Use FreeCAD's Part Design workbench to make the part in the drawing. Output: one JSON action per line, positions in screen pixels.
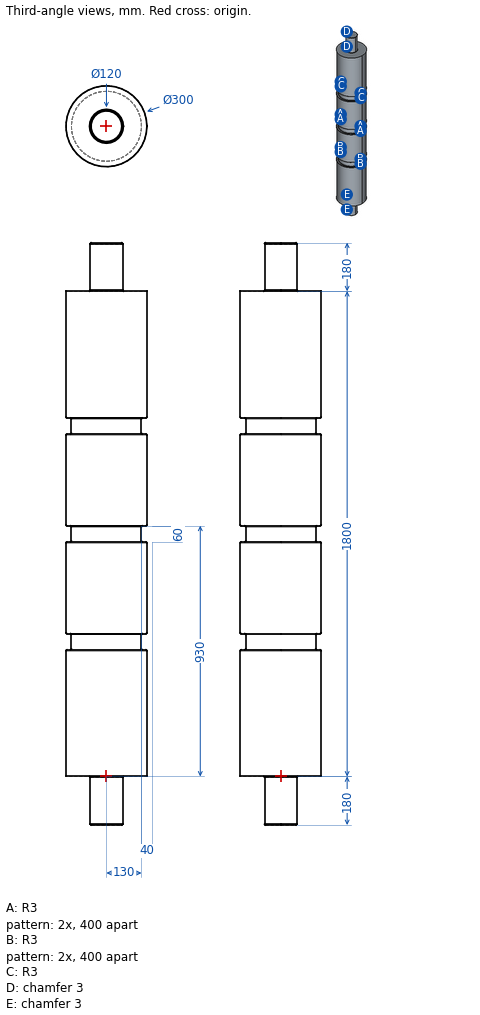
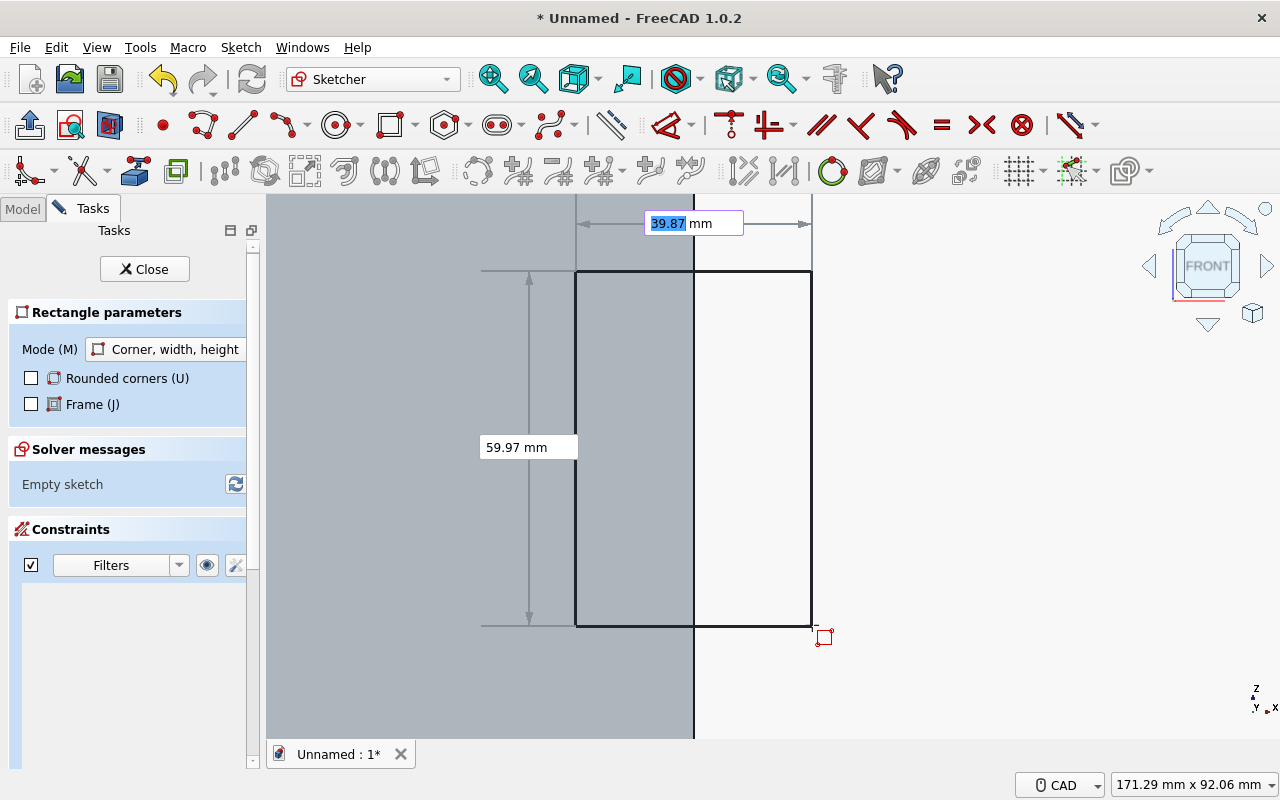
{"action": "type", "text": "40"}
{"action": "key", "text": "Tab"}
{"action": "type", "text": "60"}
{"action": "key", "text": "Return"}
{"action": "key", "text": "Escape"}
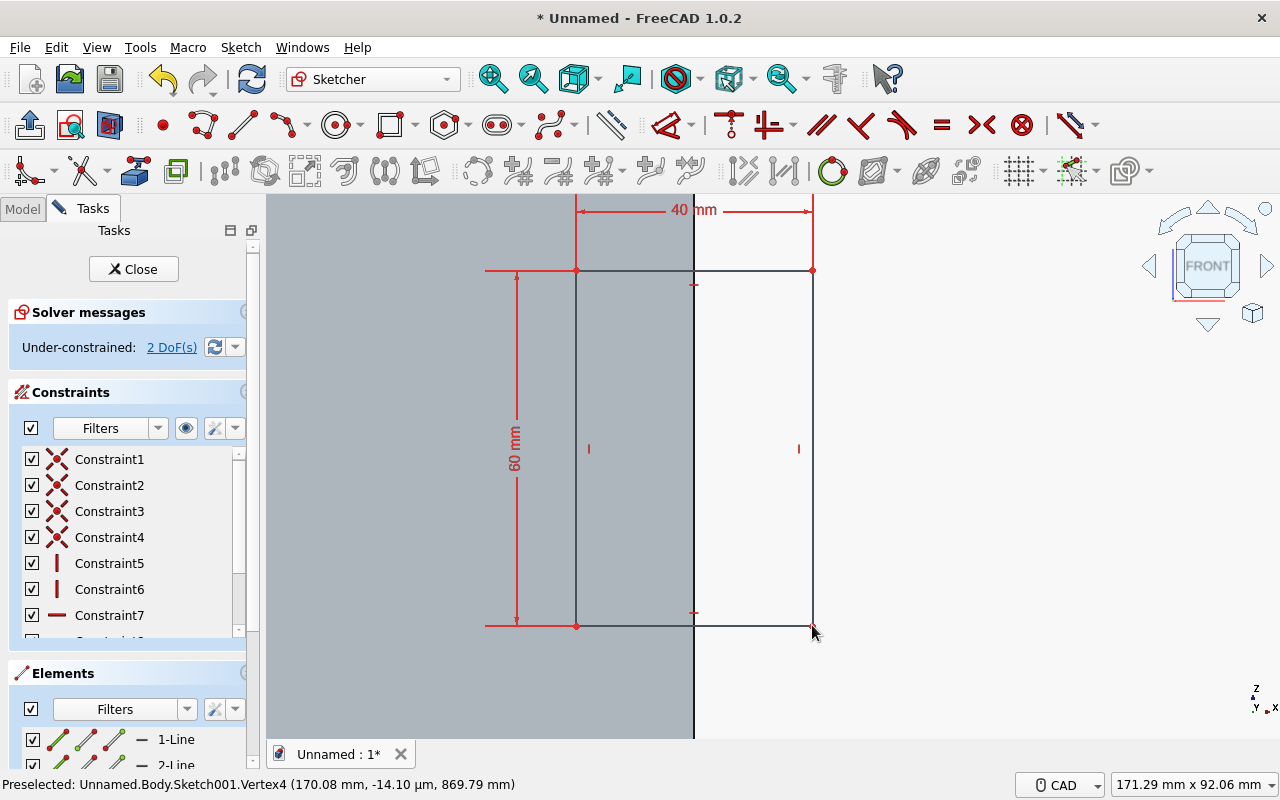
{"action": "left_click", "coordinate": [666, 126]}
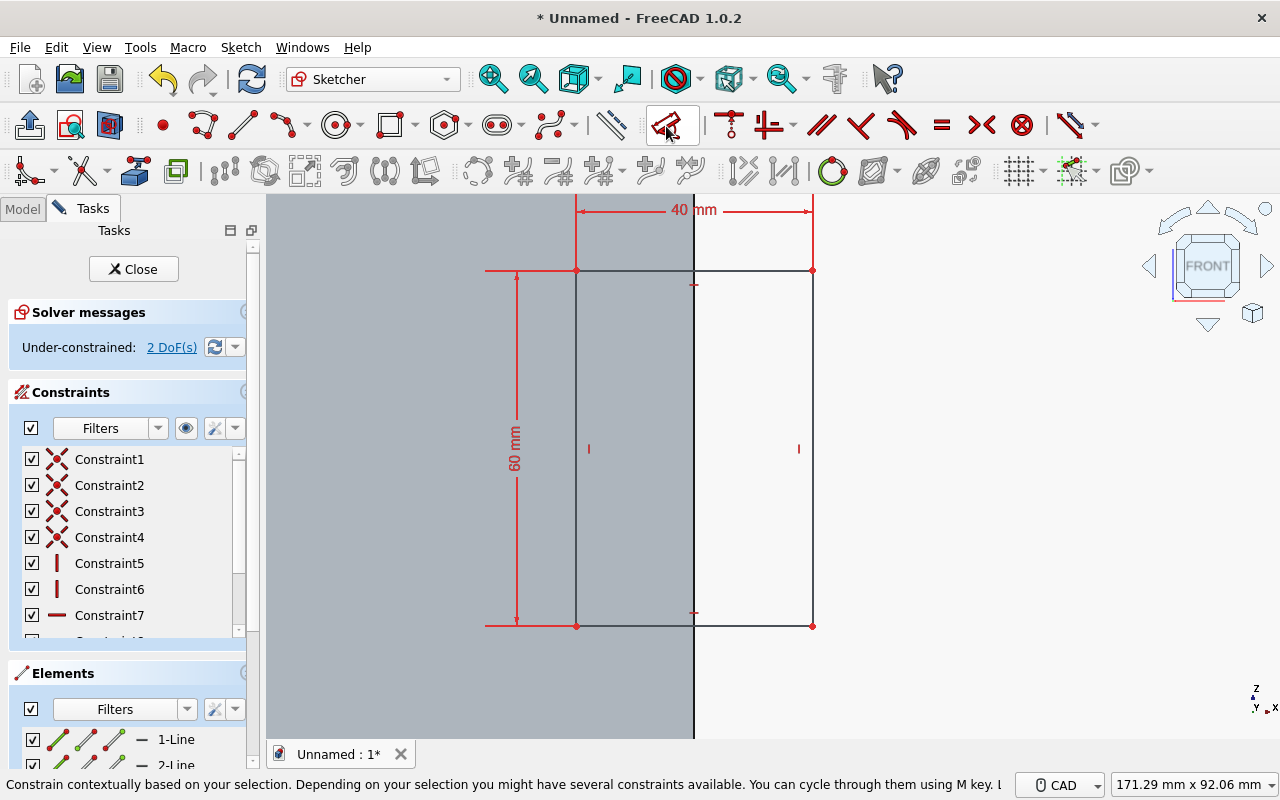
{"action": "left_click", "coordinate": [576, 271]}
{"action": "left_click", "coordinate": [435, 237]}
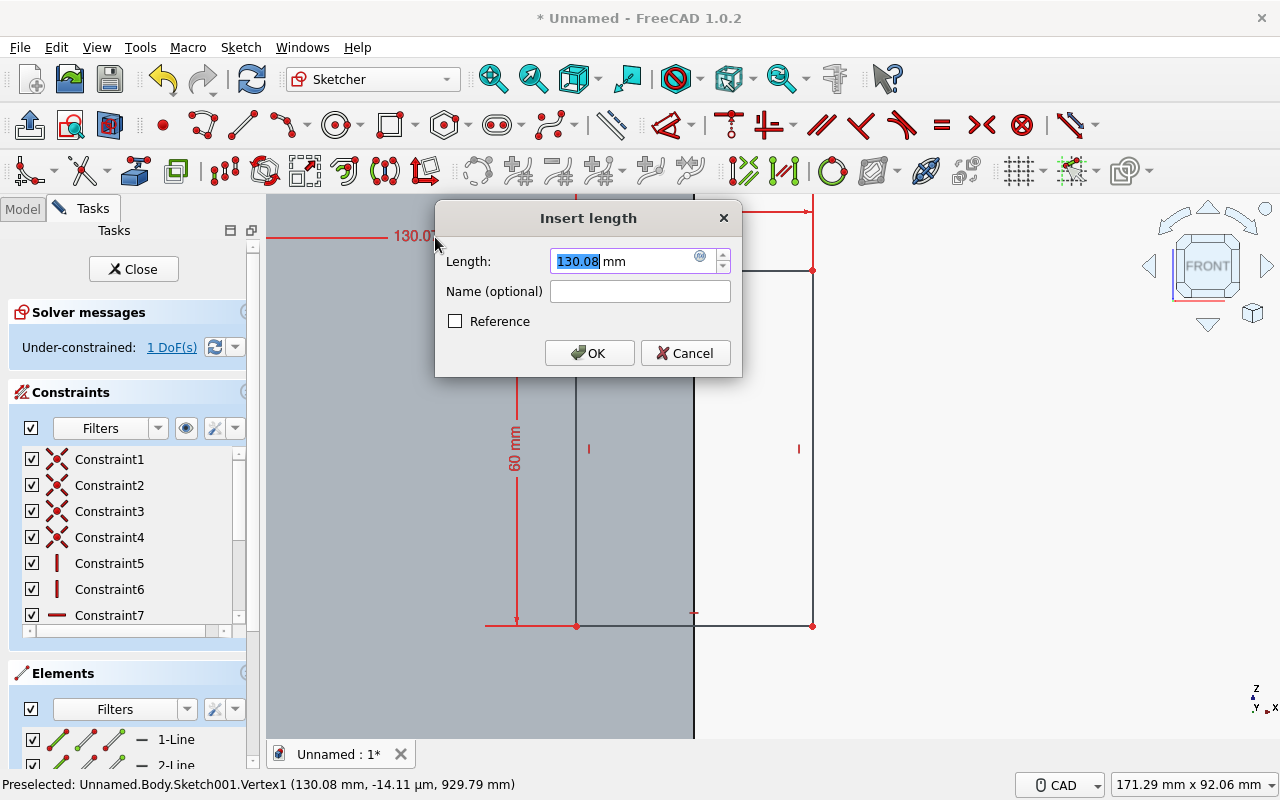
{"action": "type", "text": "130"}
{"action": "key", "text": "Return"}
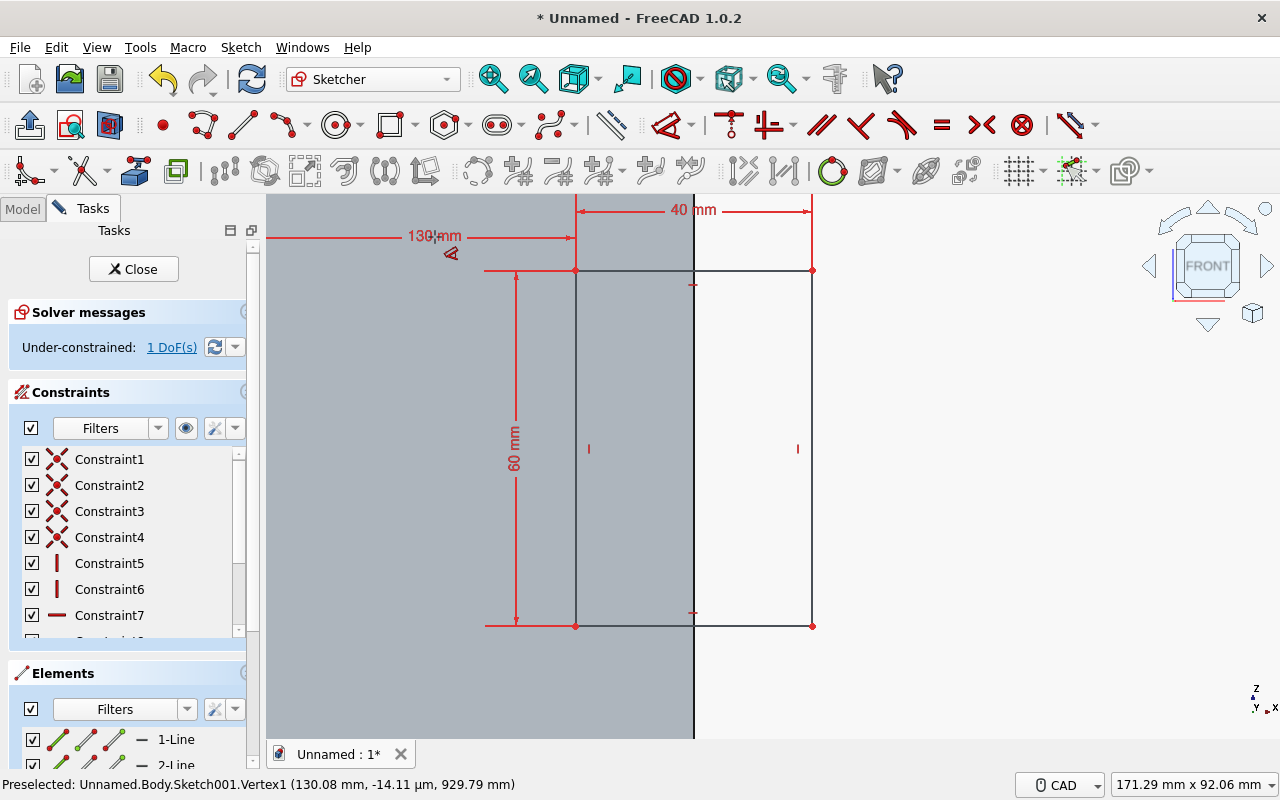
{"action": "left_click", "coordinate": [576, 271]}
{"action": "left_click", "coordinate": [610, 491]}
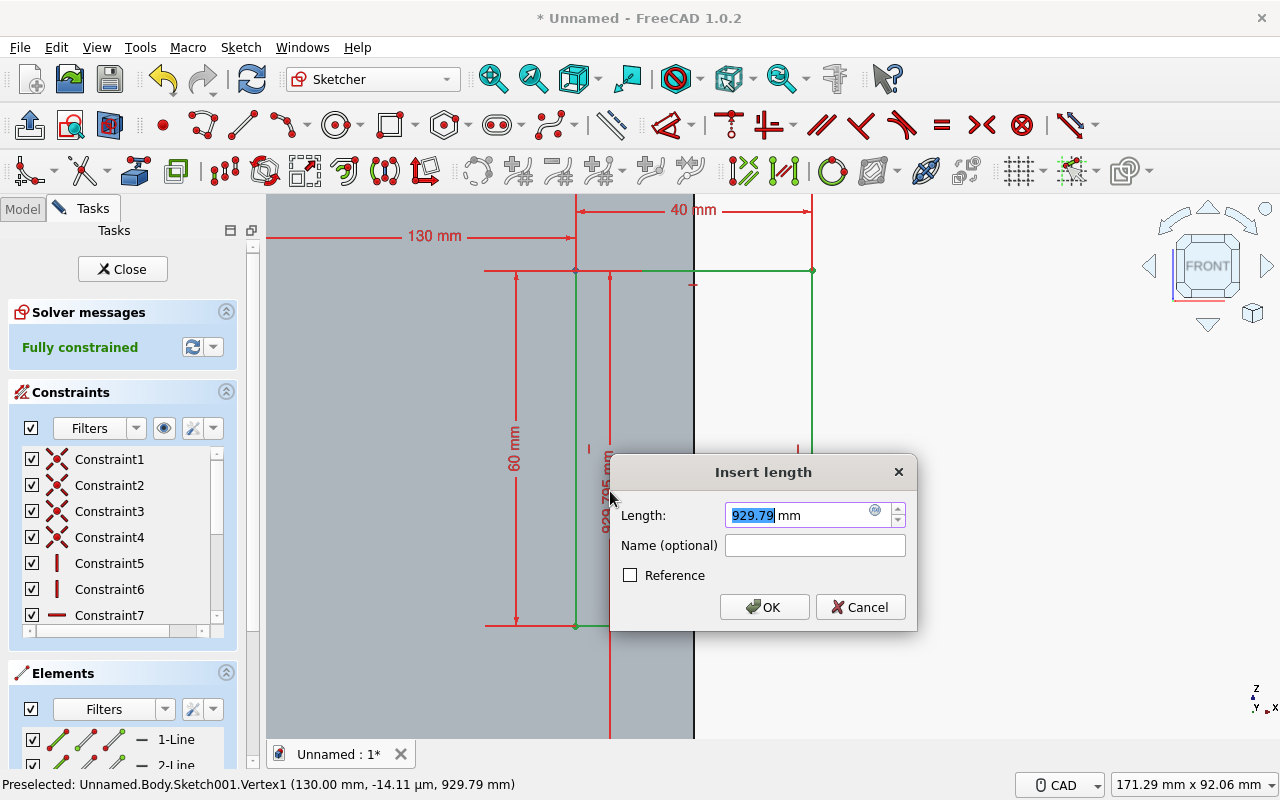
{"action": "type", "text": "930"}
{"action": "key", "text": "Return"}
{"action": "key", "text": "Escape"}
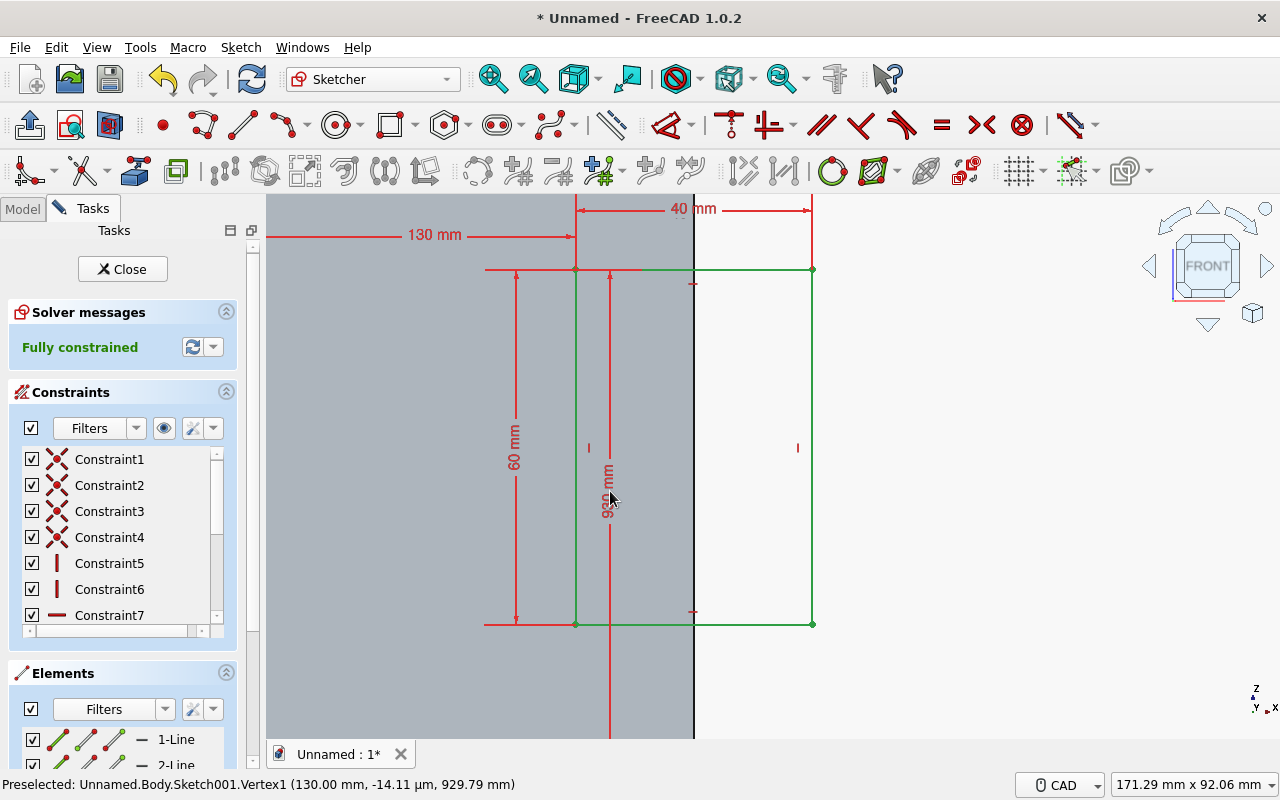
{"action": "left_click", "coordinate": [123, 269]}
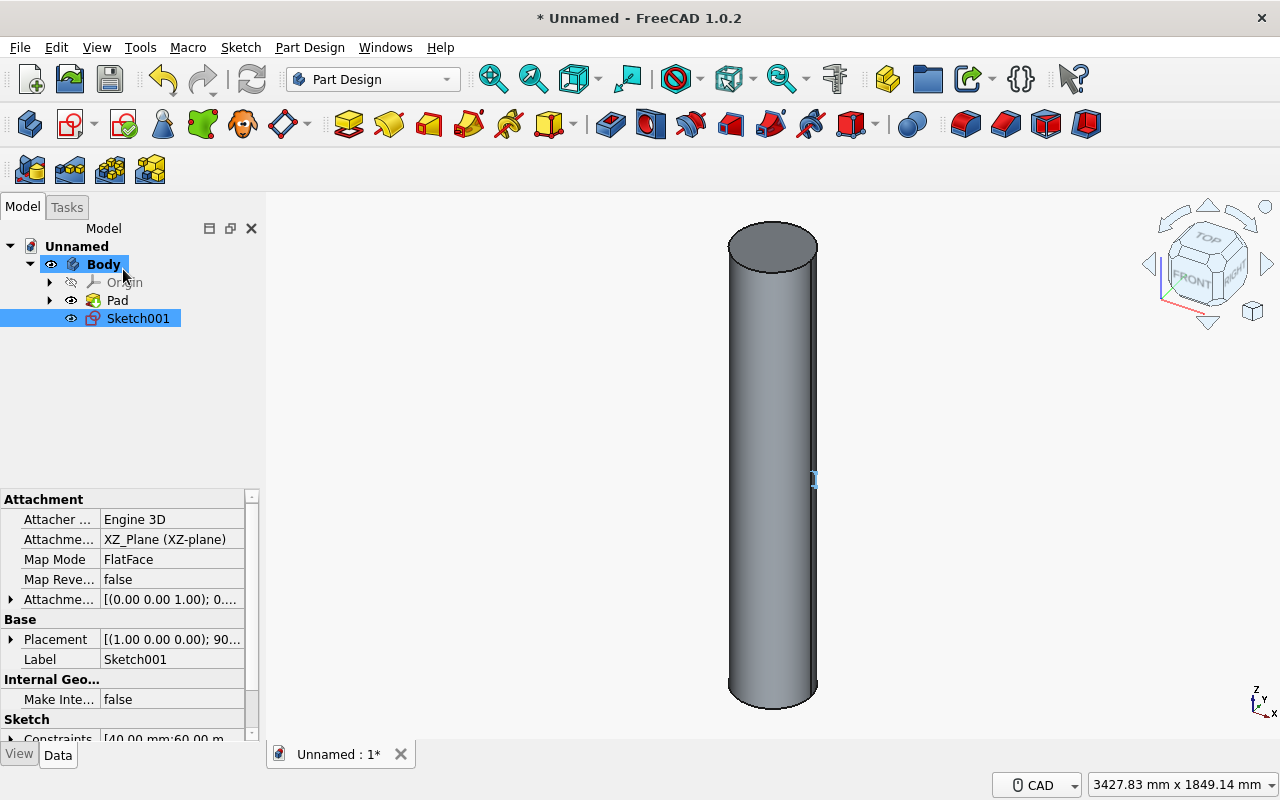
{"action": "left_click", "coordinate": [692, 124]}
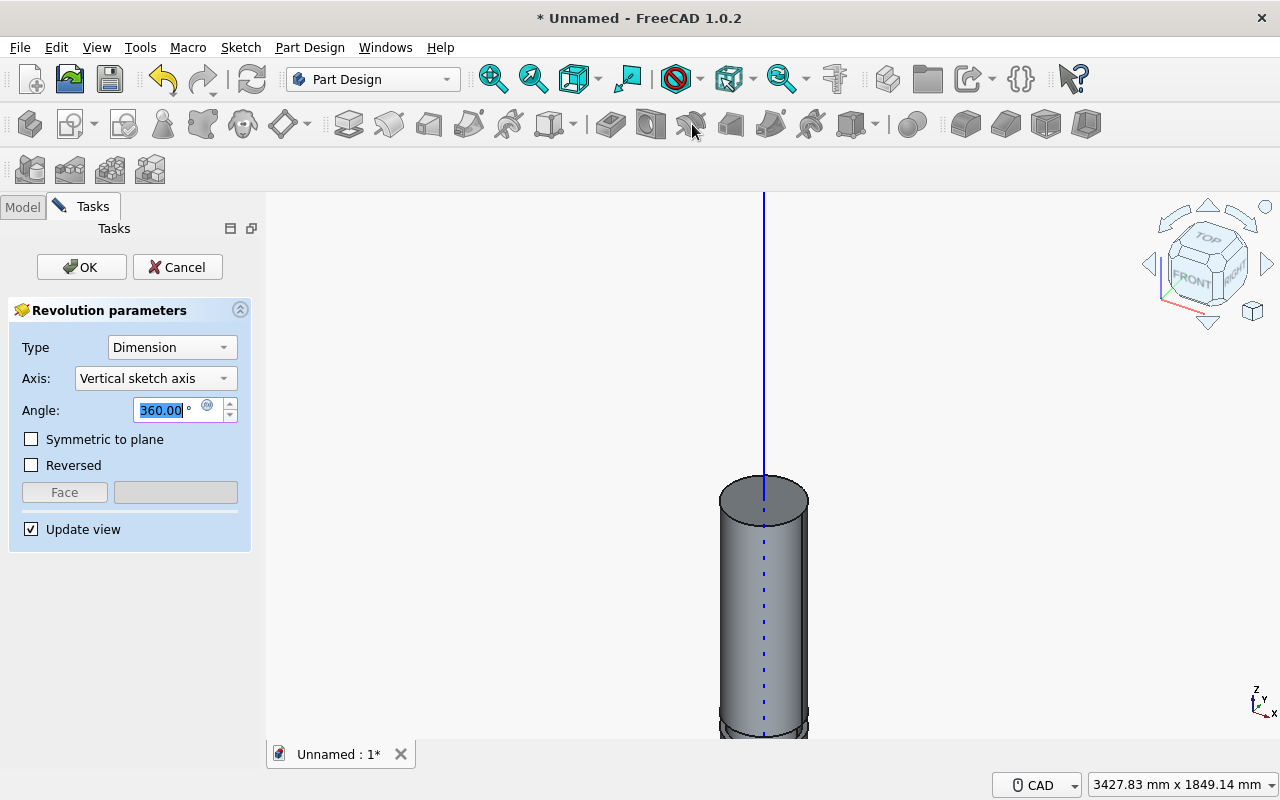
{"action": "left_click", "coordinate": [82, 267]}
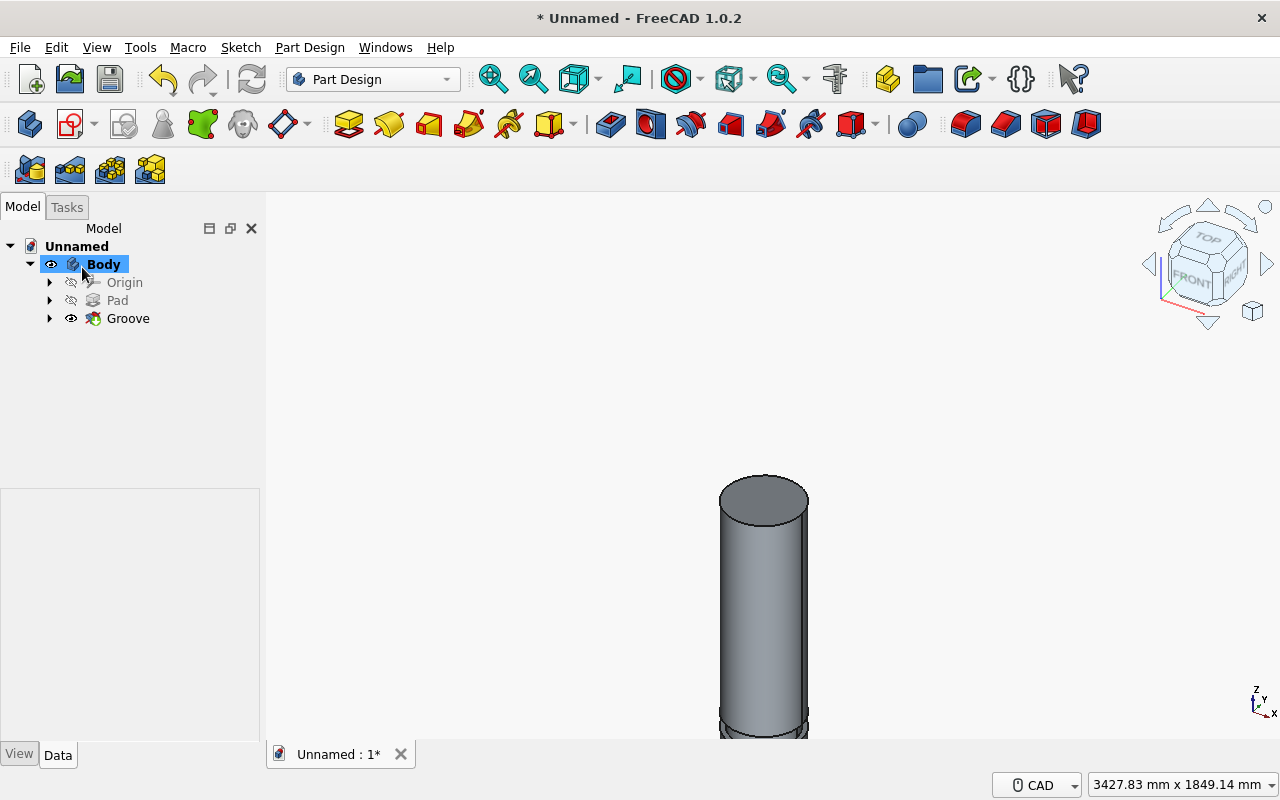
{"action": "left_click", "coordinate": [494, 80]}